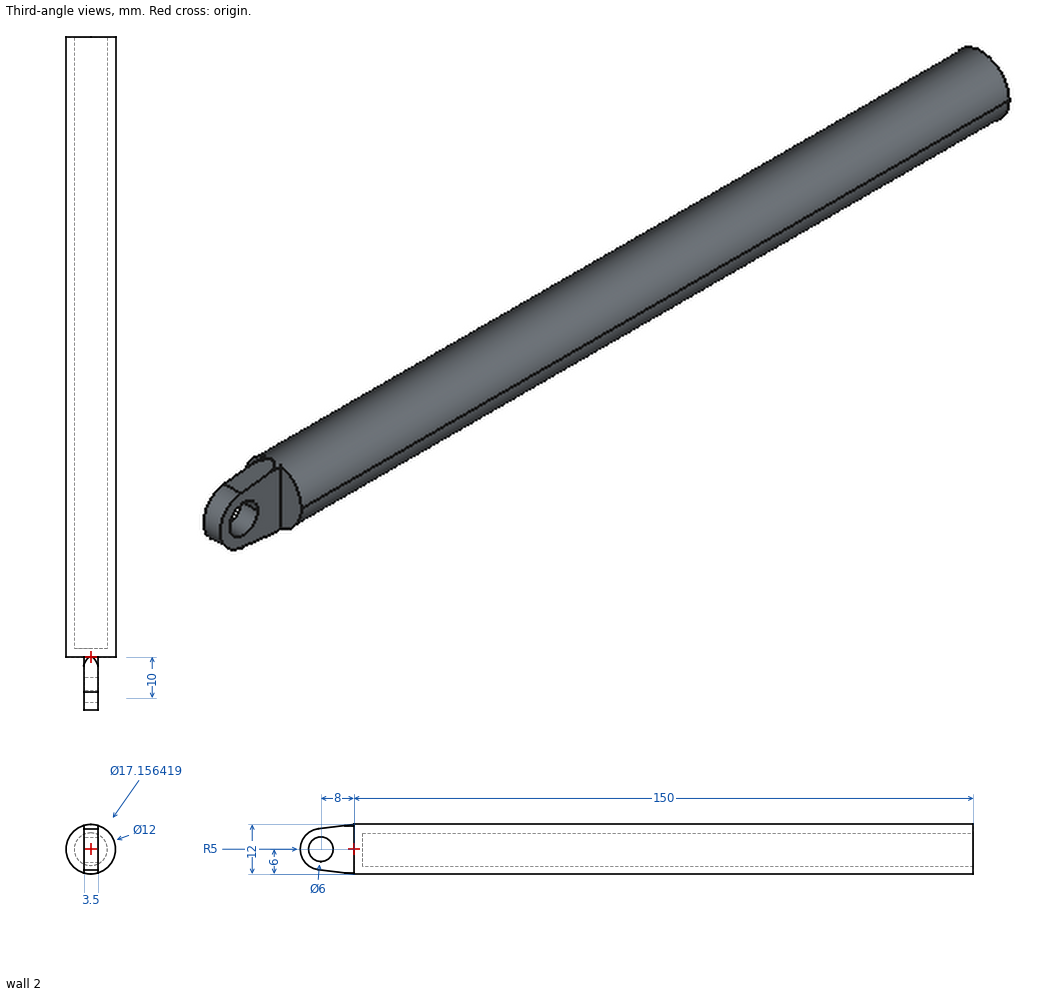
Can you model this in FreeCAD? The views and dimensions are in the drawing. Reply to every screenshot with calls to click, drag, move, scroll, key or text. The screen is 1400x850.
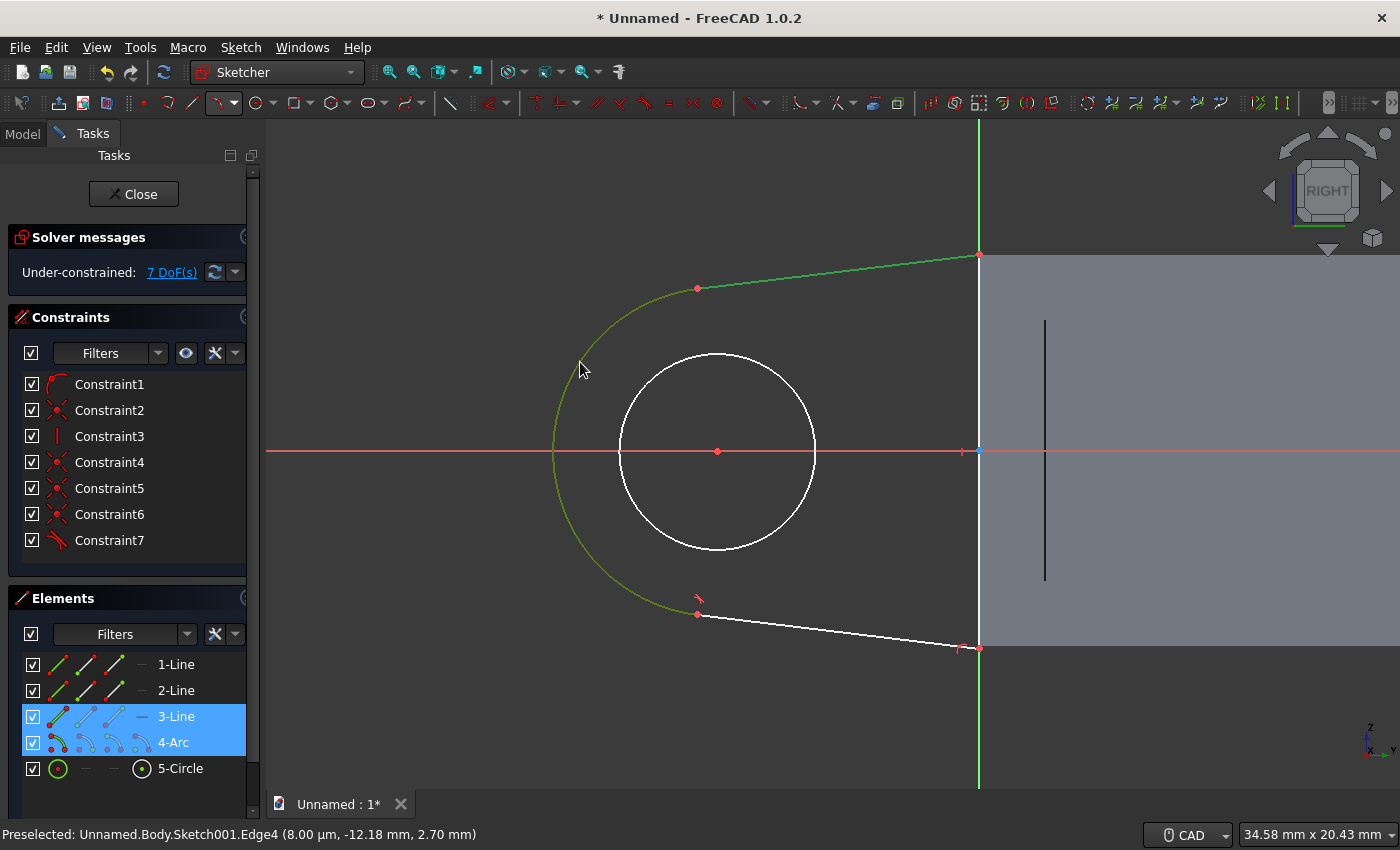
click(646, 104)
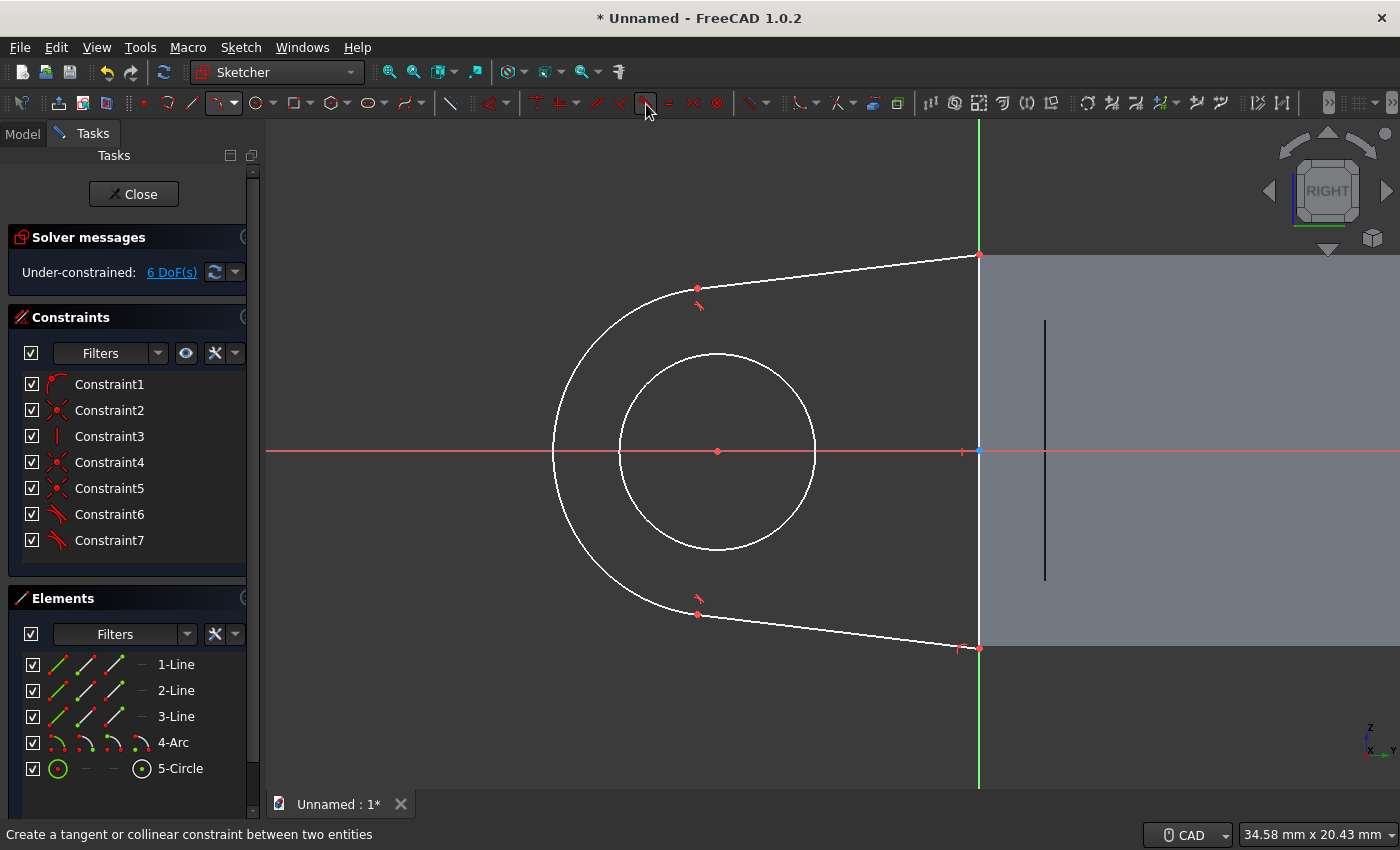
click(717, 452)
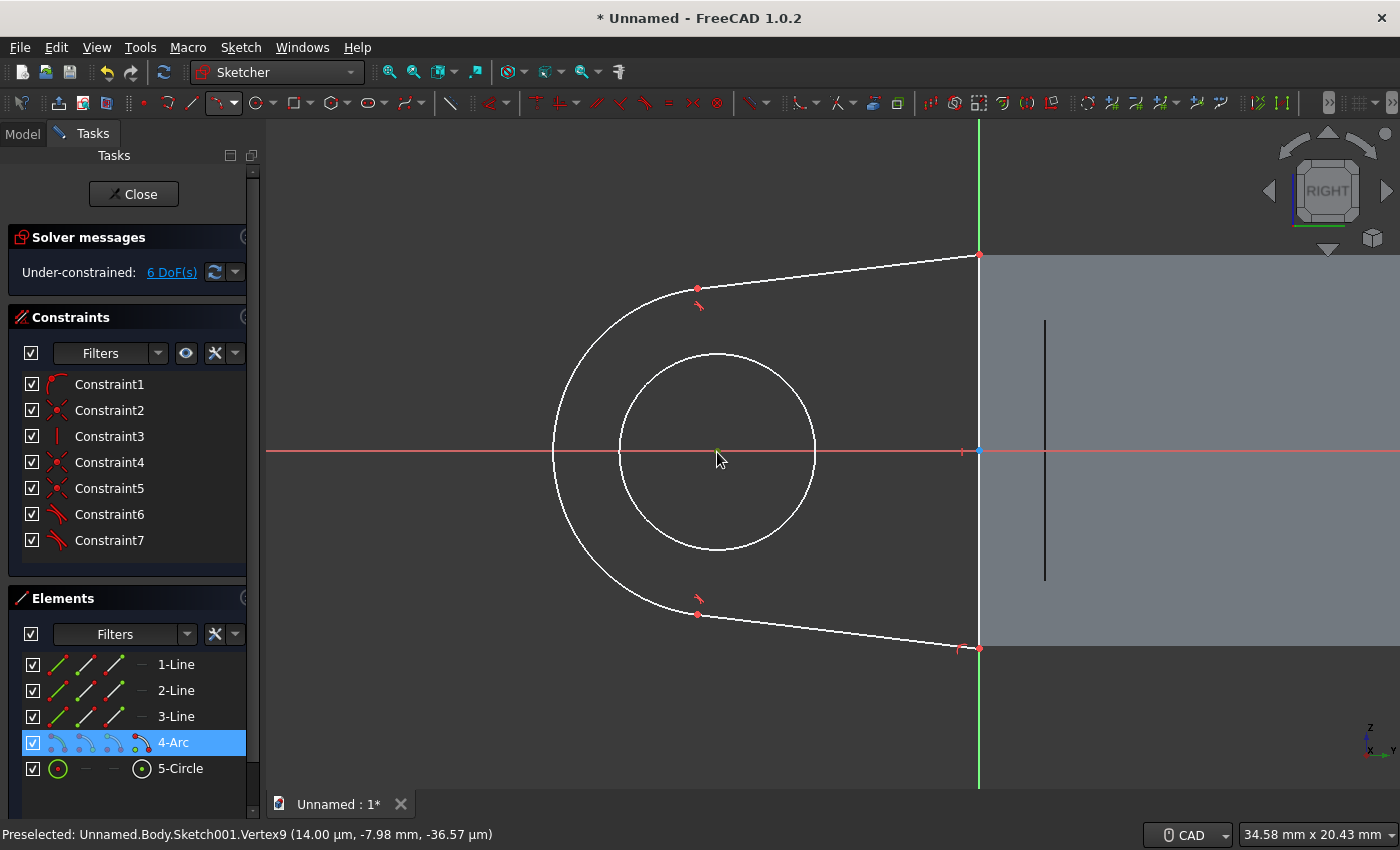
click(361, 451)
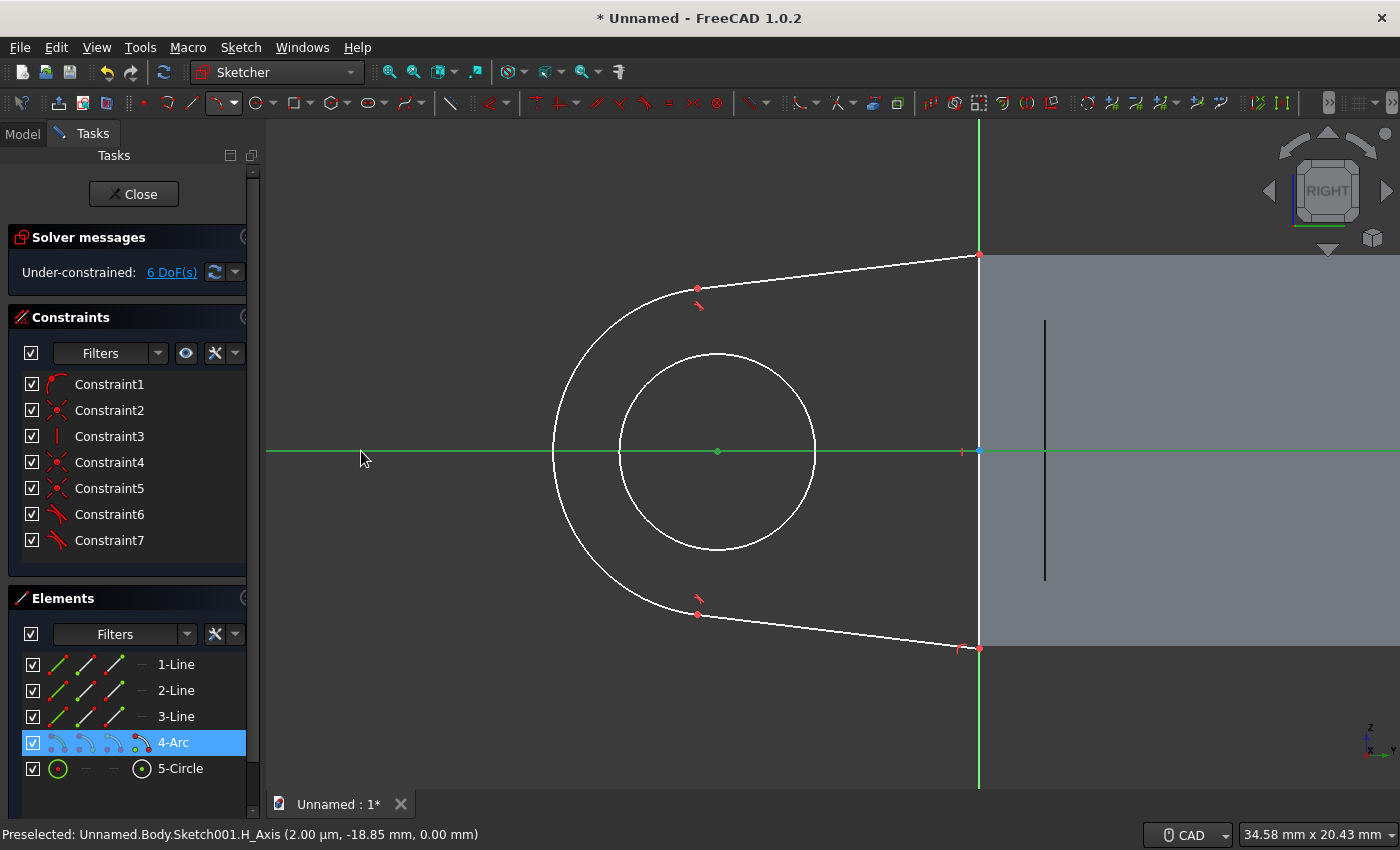
click(536, 104)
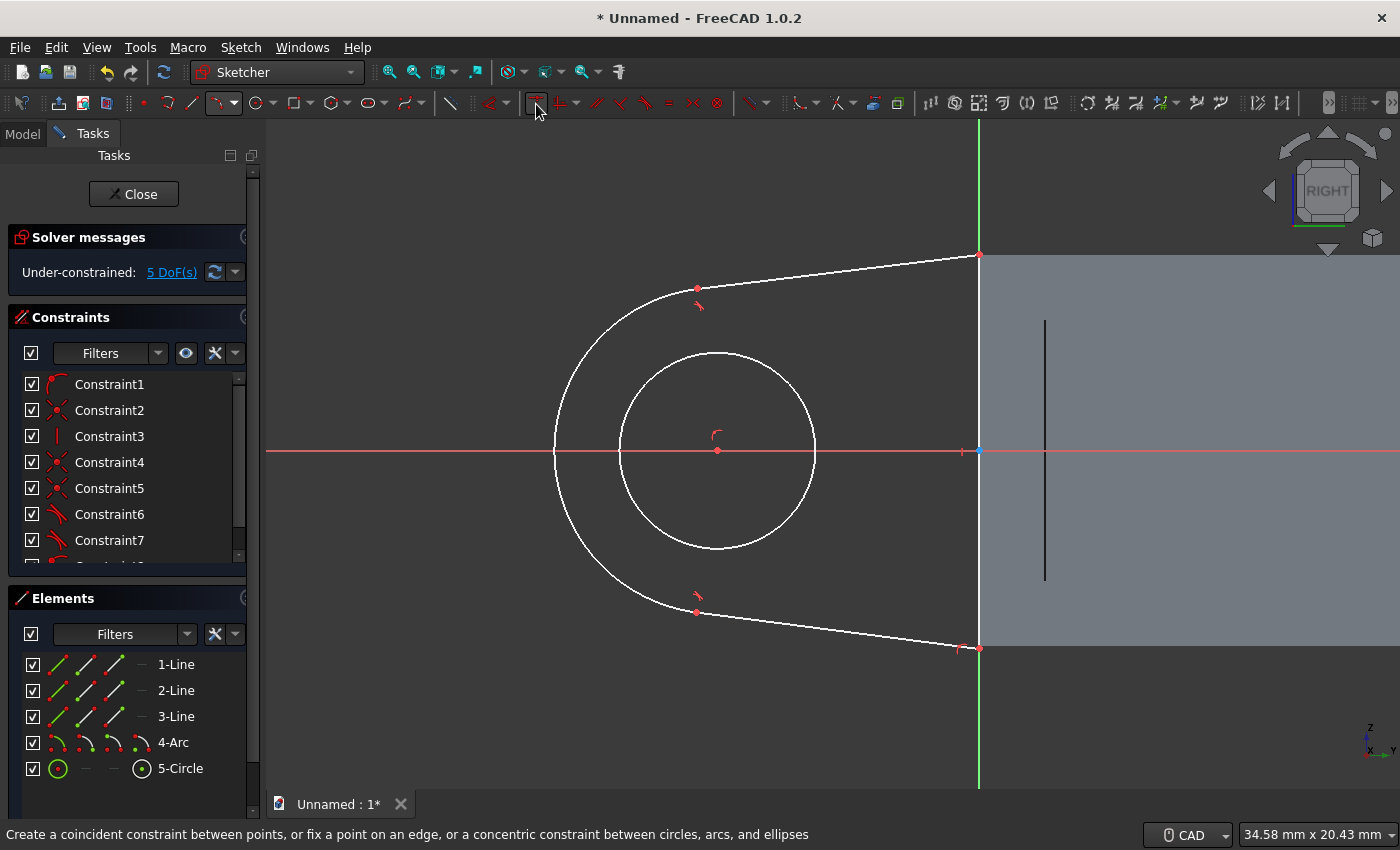
click(490, 104)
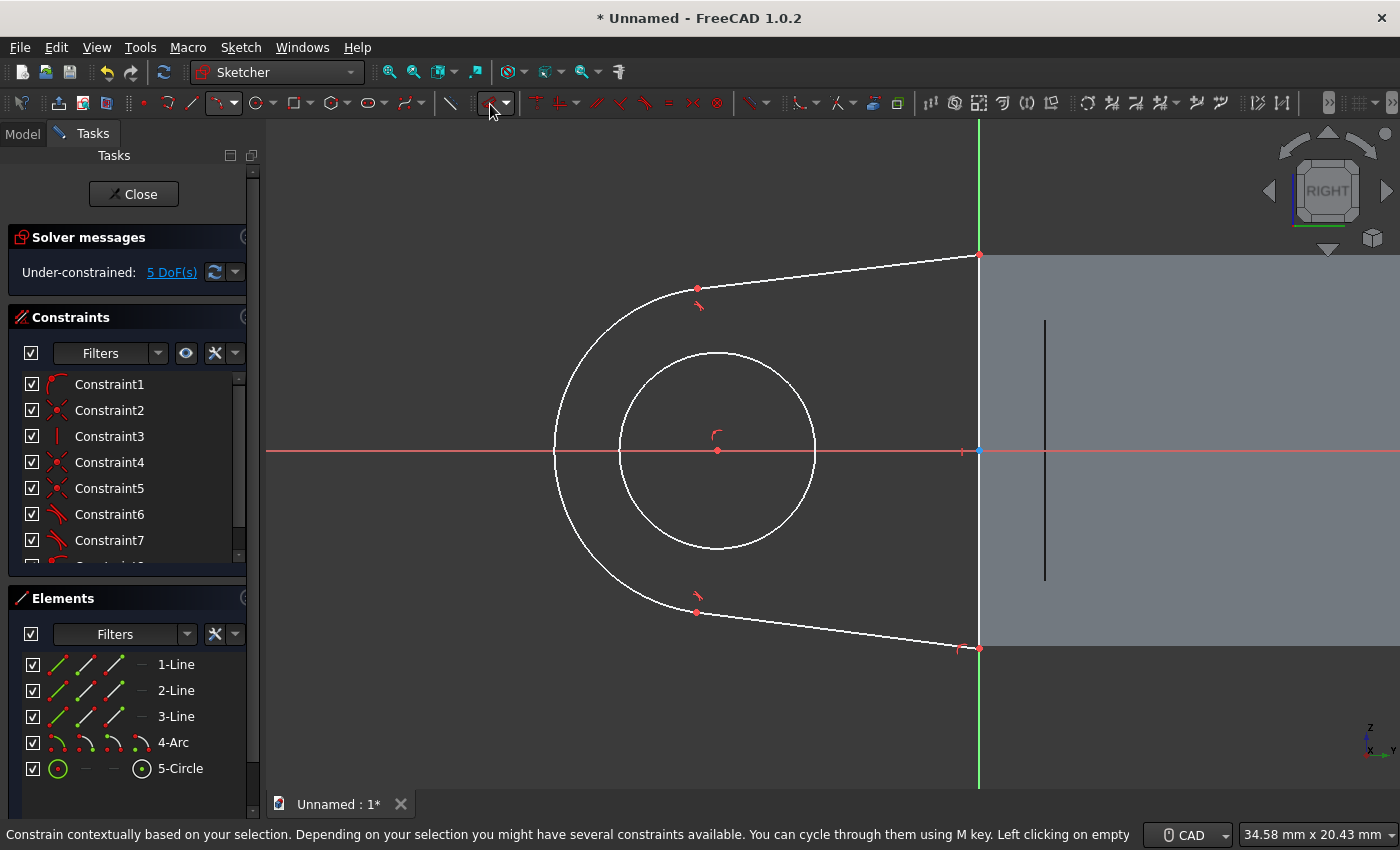
click(581, 361)
click(554, 343)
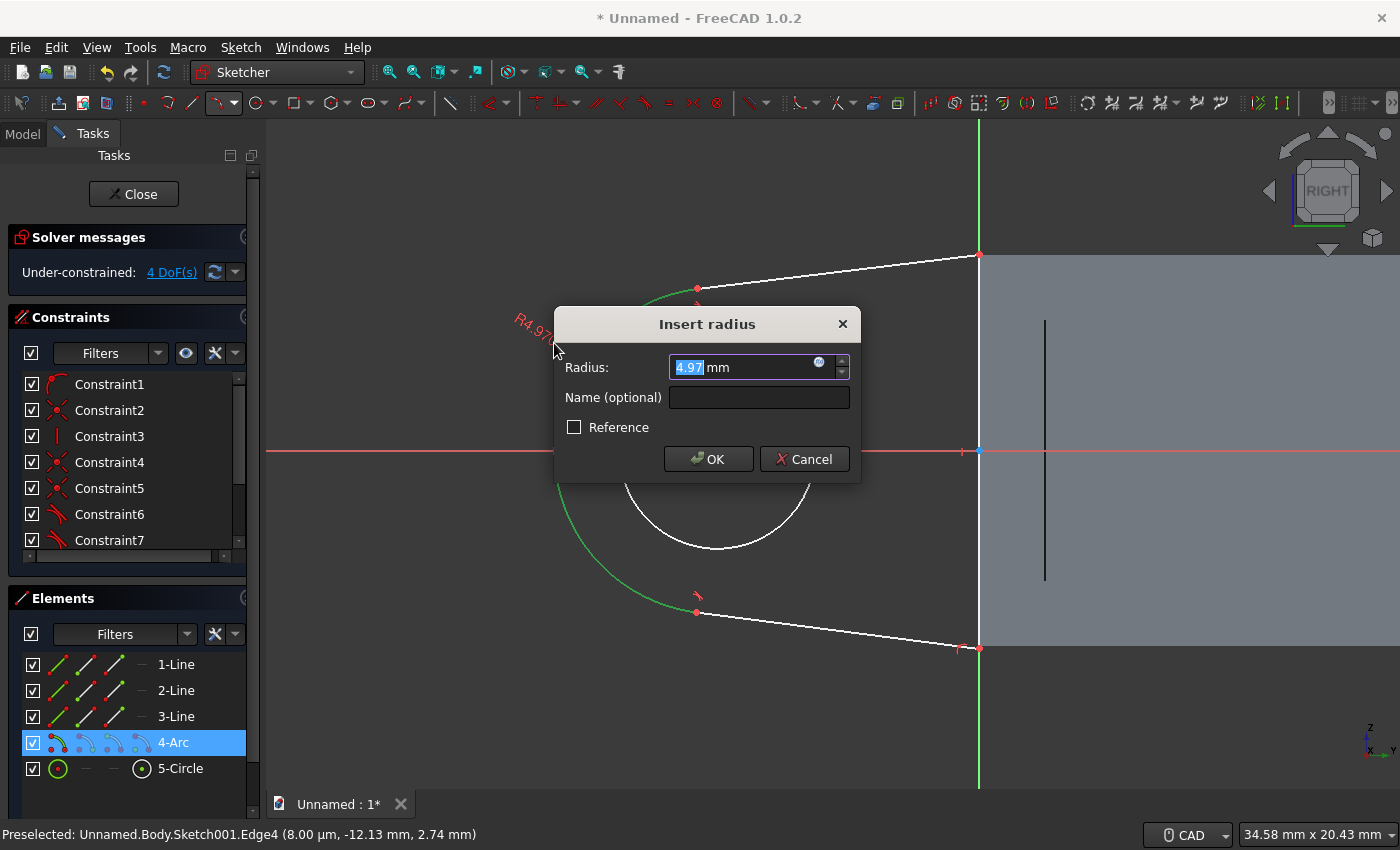
text(5)
key(Return)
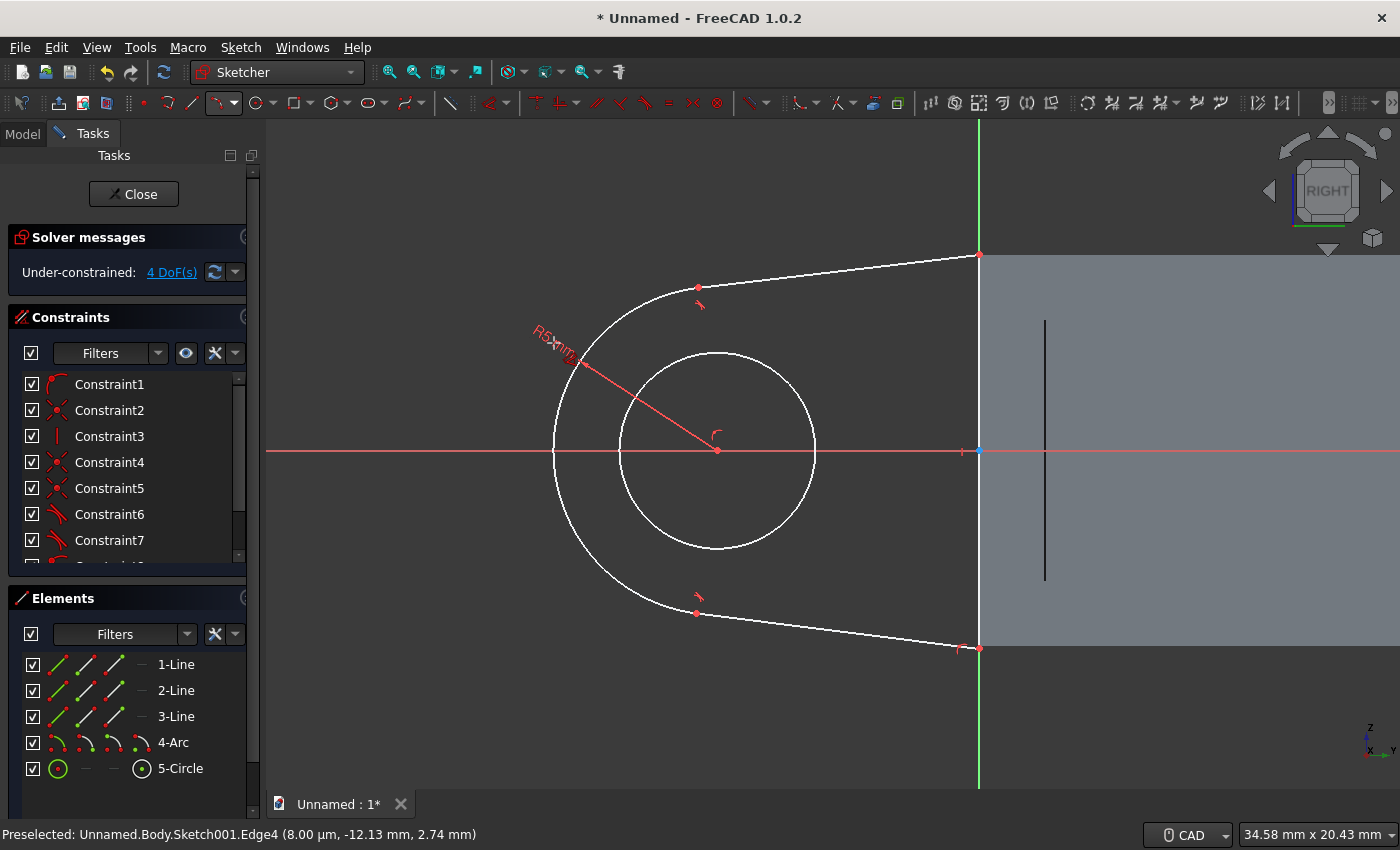
click(786, 381)
click(808, 358)